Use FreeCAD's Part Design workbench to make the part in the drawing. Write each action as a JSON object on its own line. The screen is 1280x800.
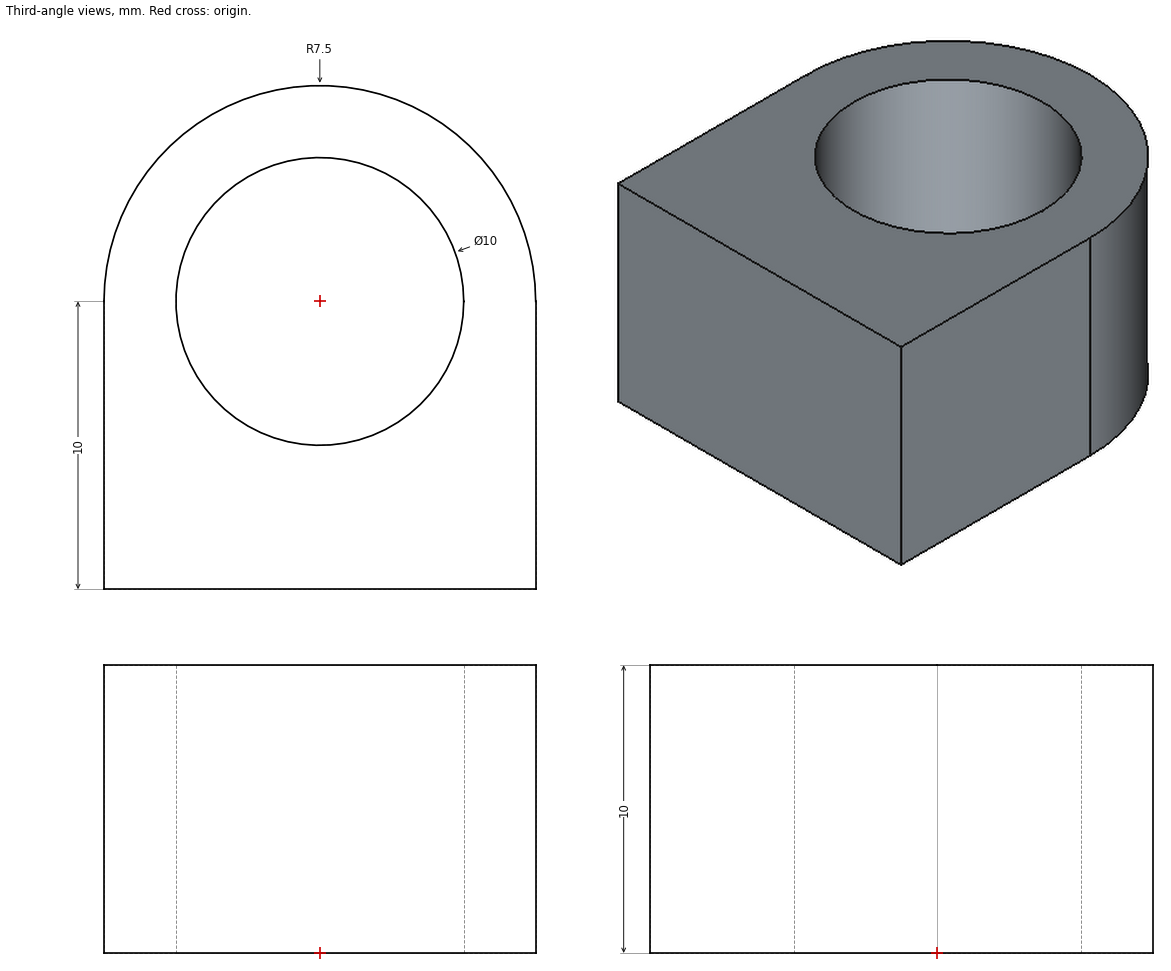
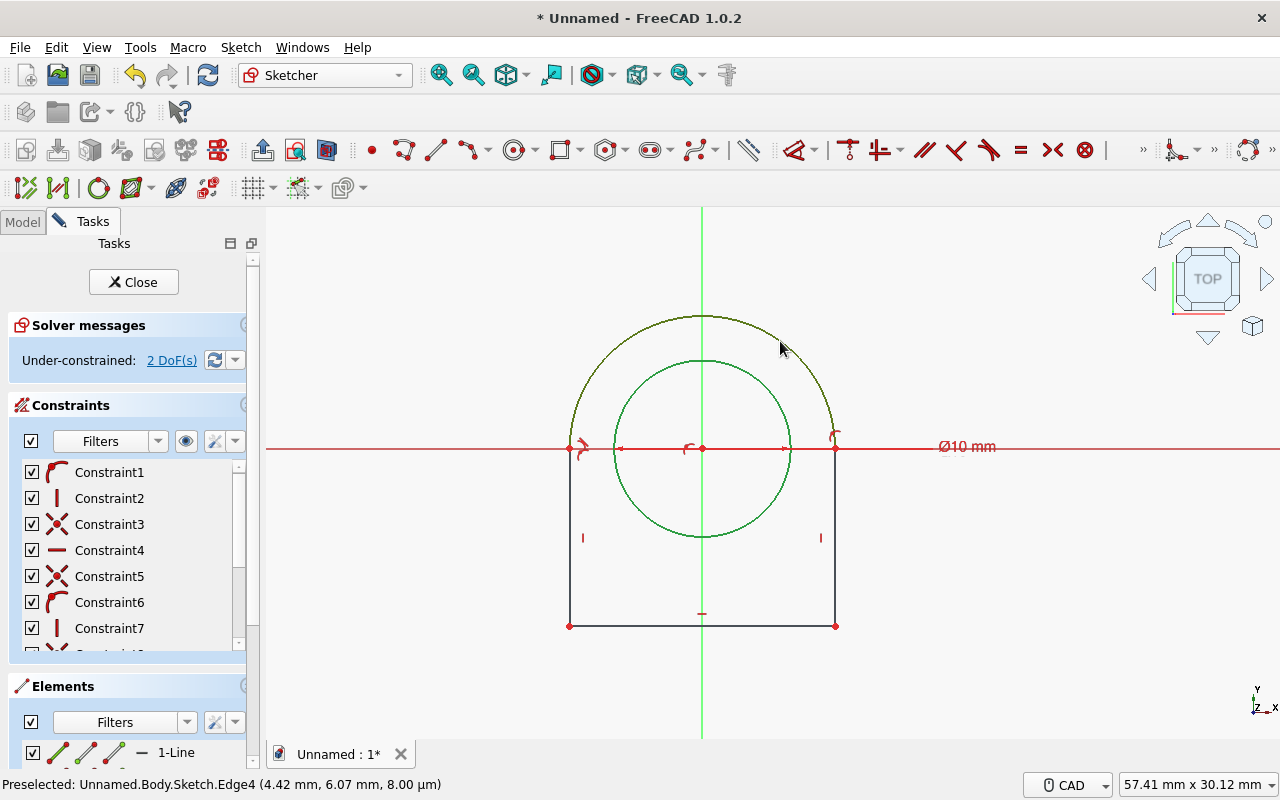
{"action": "left_click", "coordinate": [816, 150]}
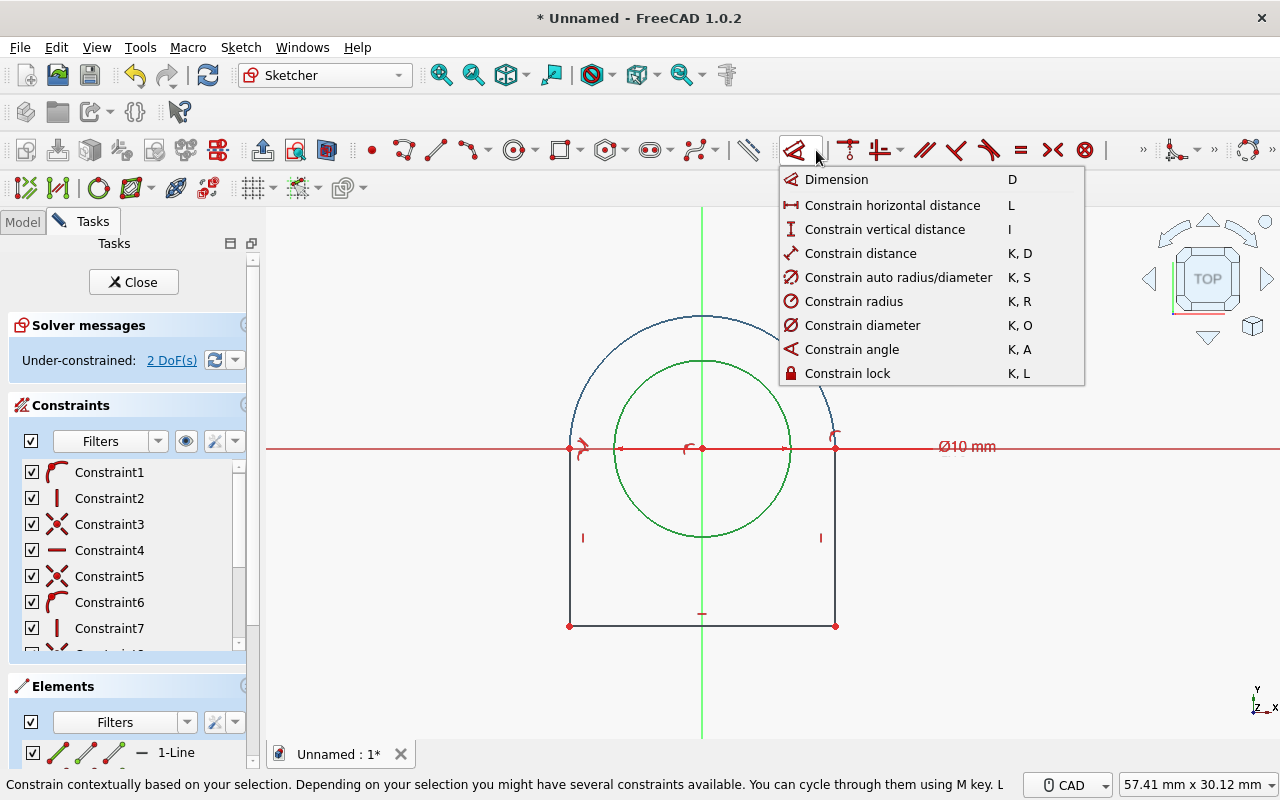
{"action": "left_click", "coordinate": [932, 301]}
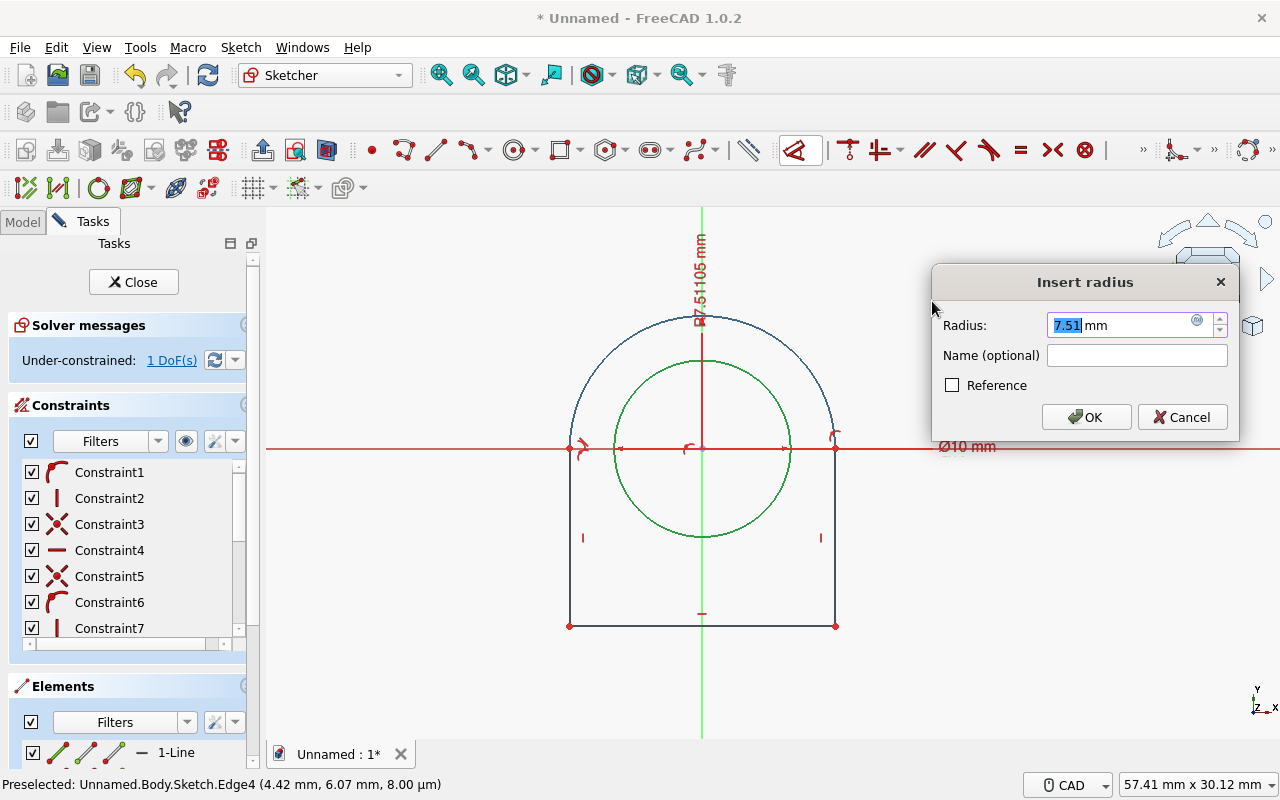
{"action": "type", "text": "7.5"}
{"action": "key", "text": "Return"}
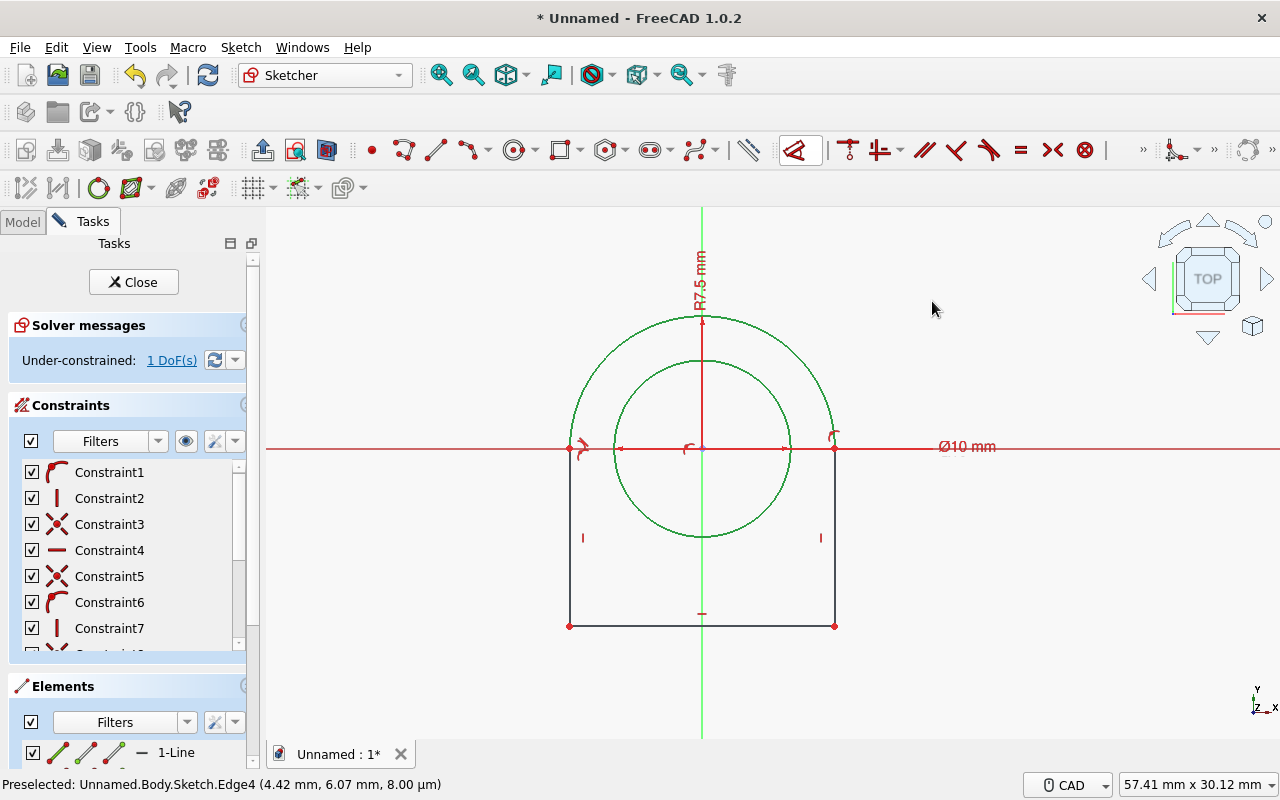
{"action": "left_click", "coordinate": [570, 502]}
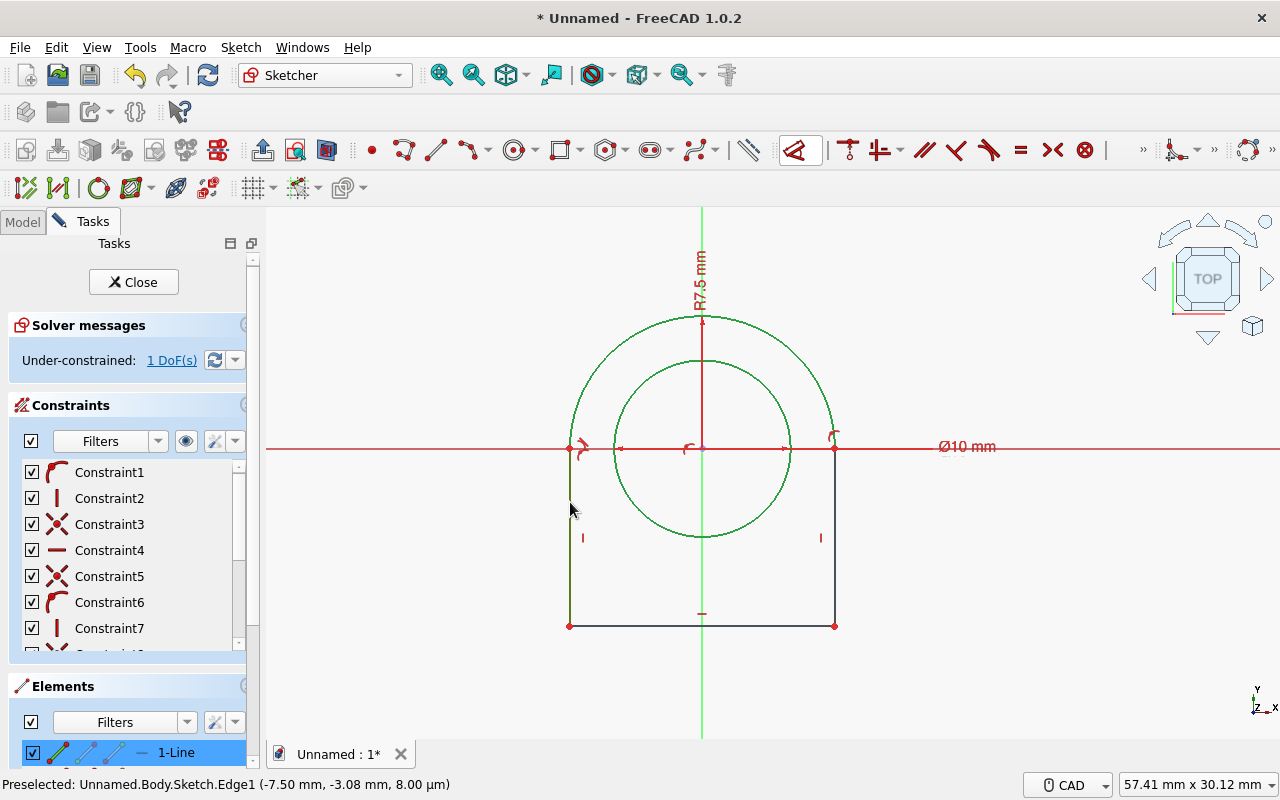
{"action": "key", "text": "i"}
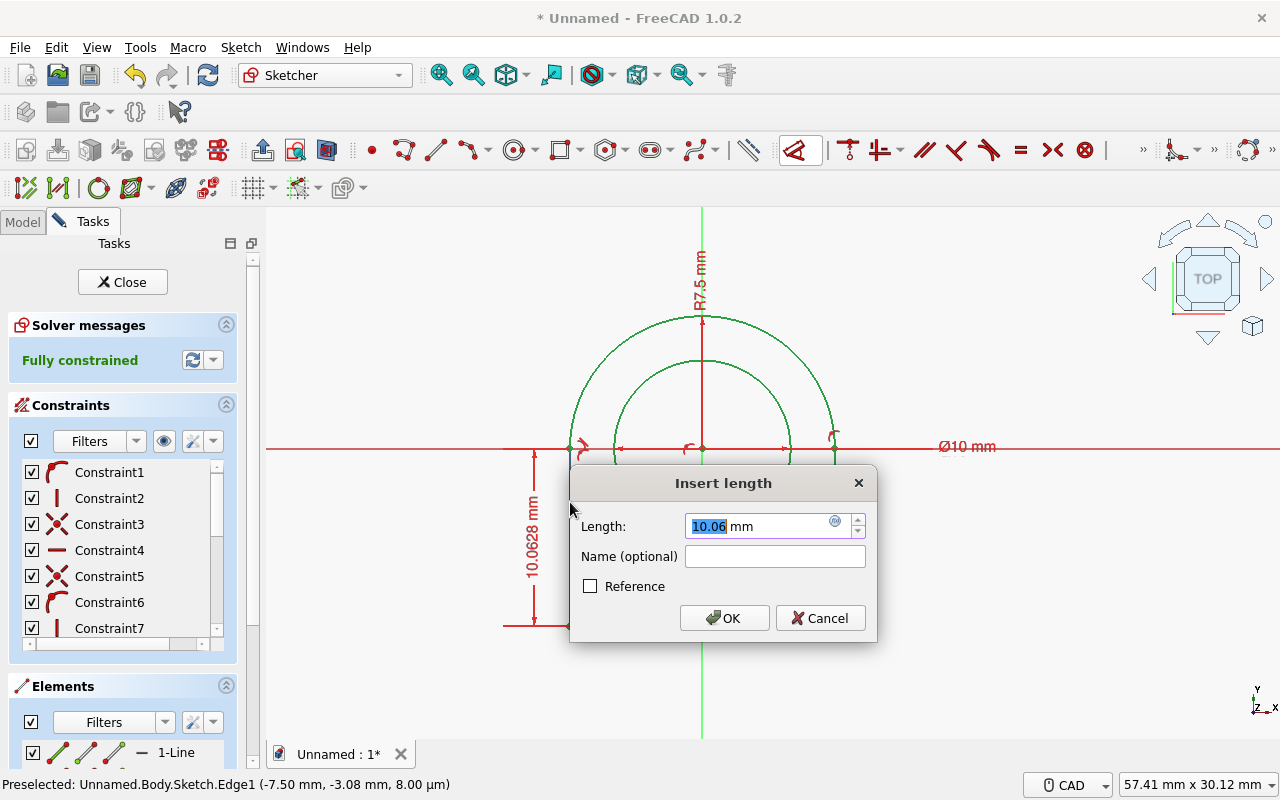
{"action": "type", "text": "10"}
{"action": "key", "text": "Return"}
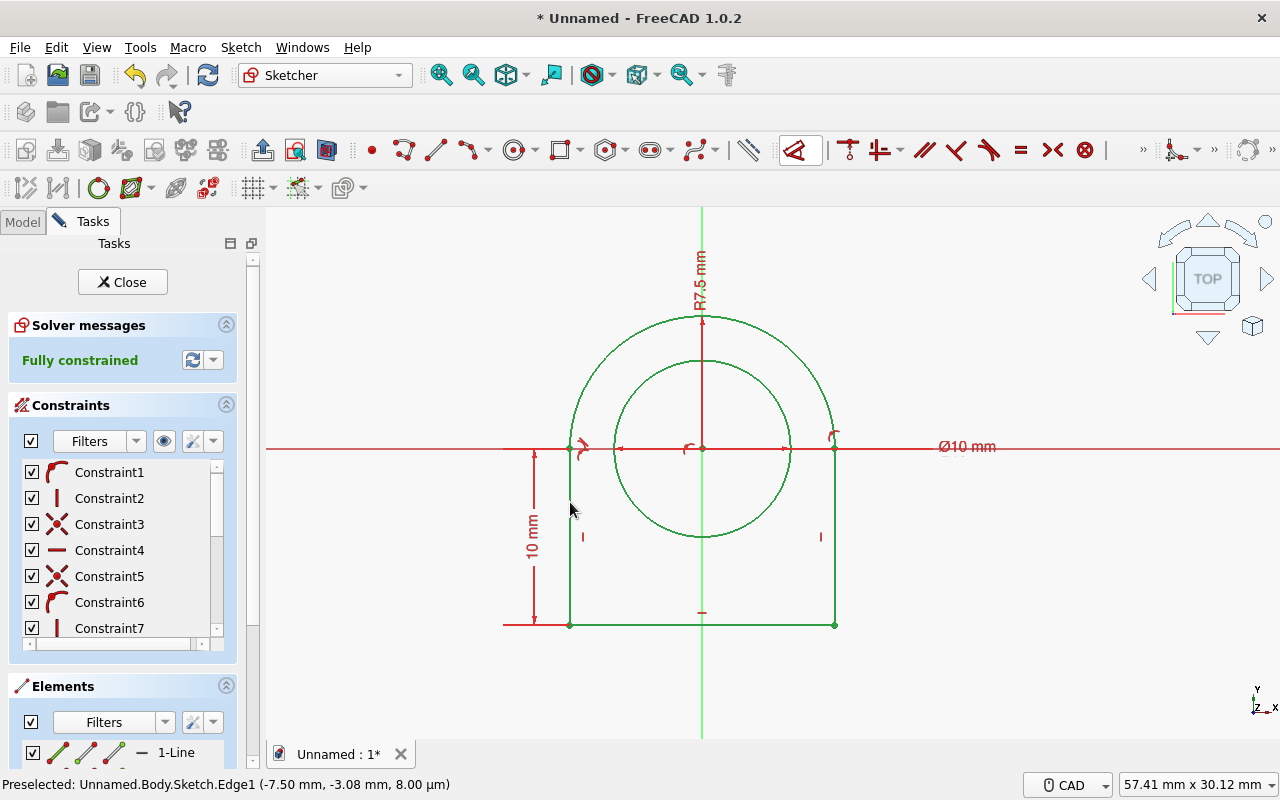
{"action": "left_click", "coordinate": [123, 282]}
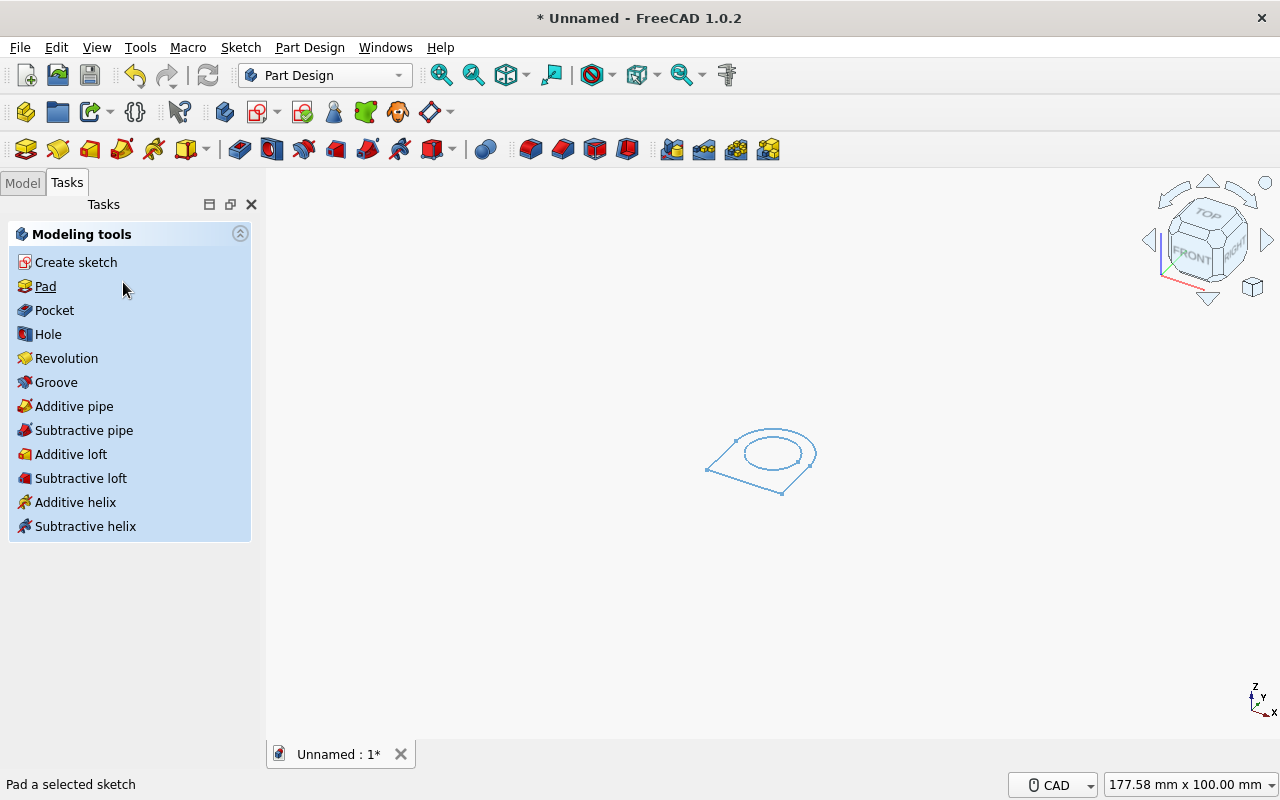
{"action": "left_click", "coordinate": [26, 150]}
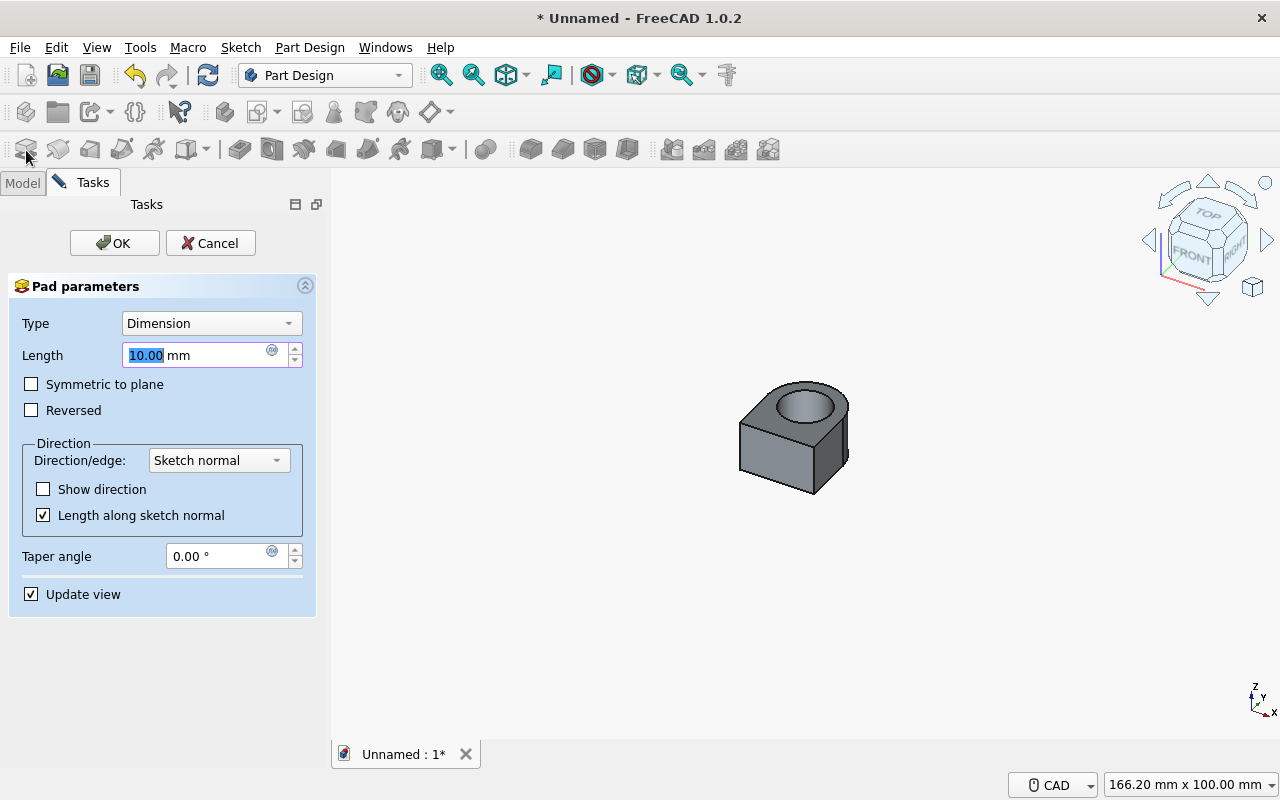
{"action": "type", "text": "10"}
{"action": "key", "text": "Tab"}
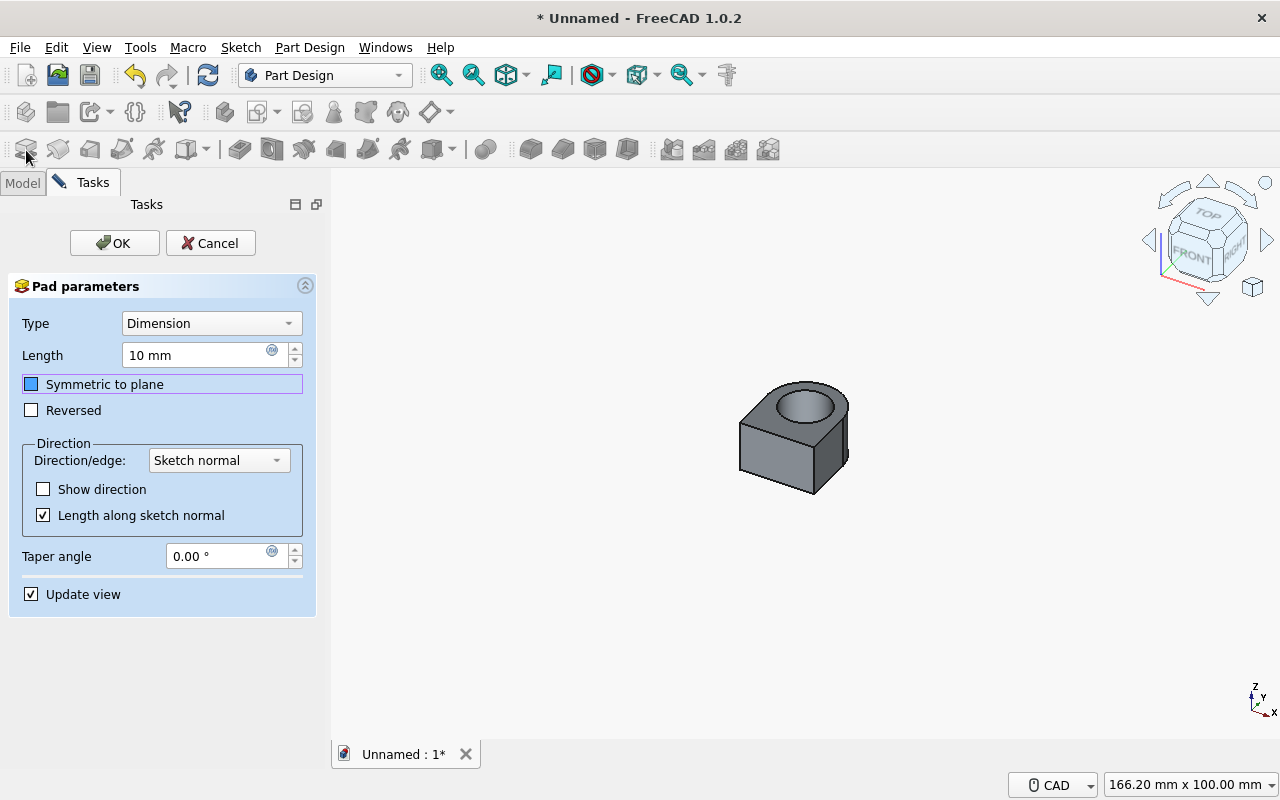
{"action": "left_click", "coordinate": [115, 243]}